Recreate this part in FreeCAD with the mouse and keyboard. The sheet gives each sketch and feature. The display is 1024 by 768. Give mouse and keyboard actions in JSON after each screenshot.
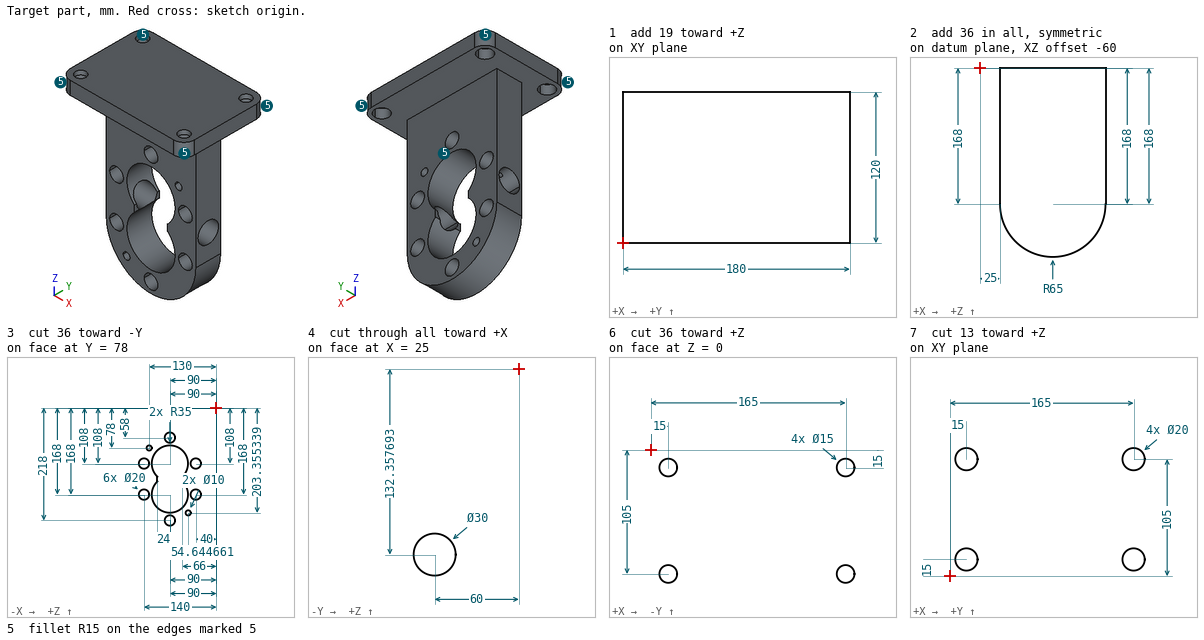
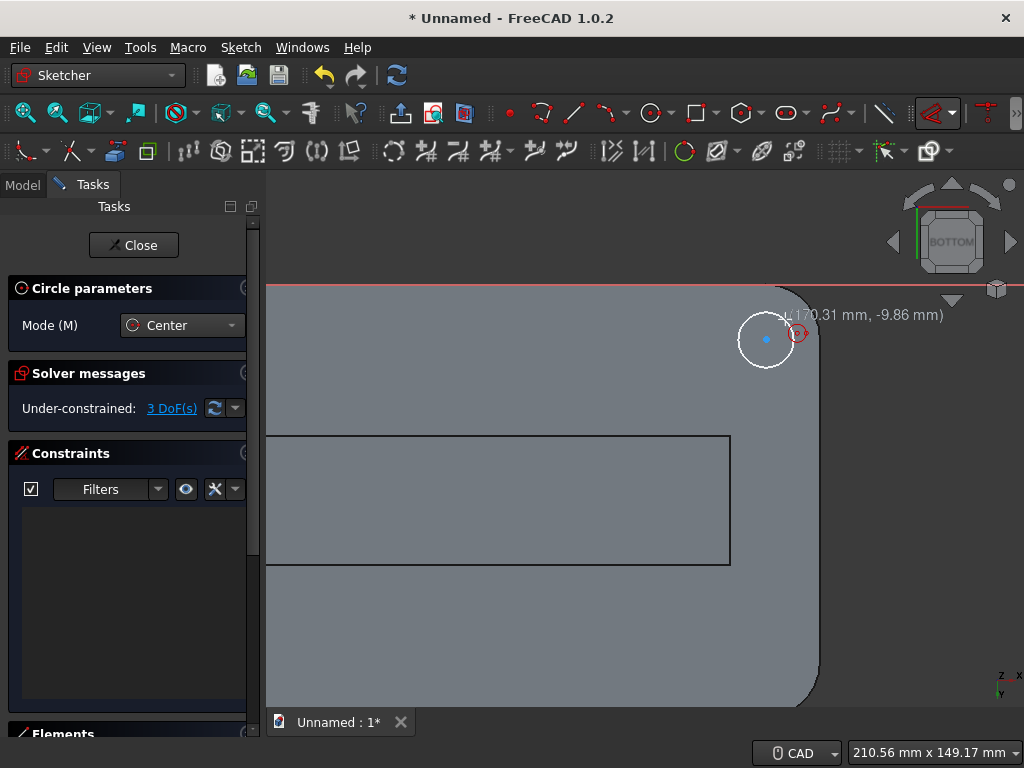
{"action": "scroll", "coordinate": [768, 340], "scroll_direction": "down", "scroll_amount": 2}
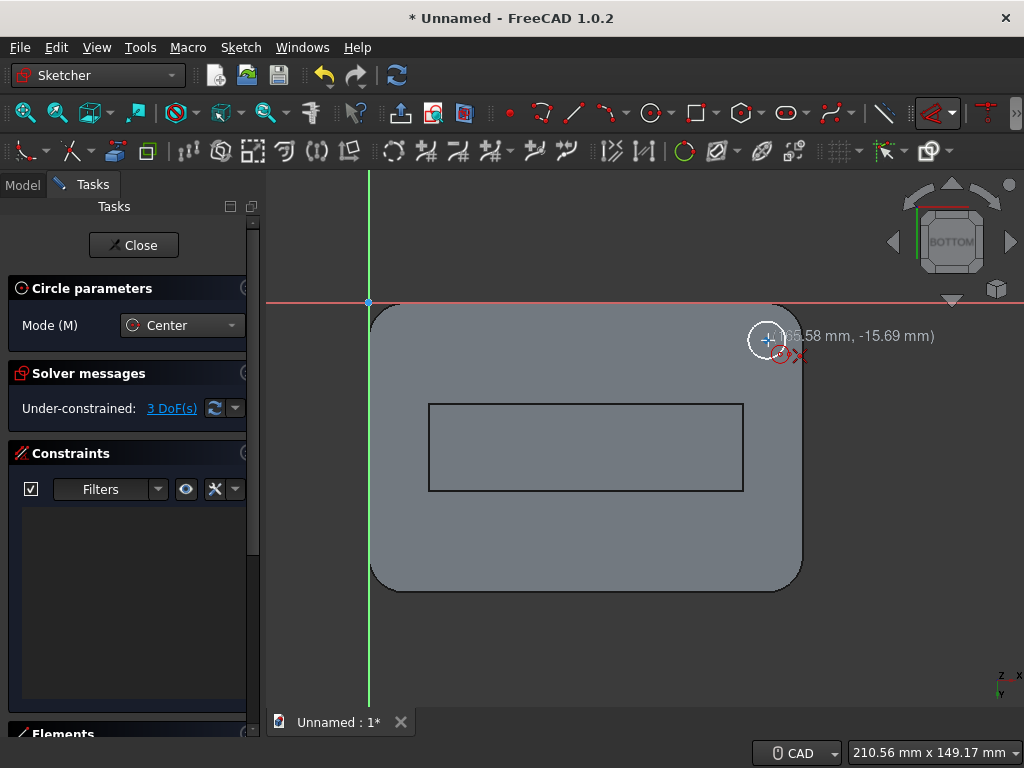
{"action": "scroll", "coordinate": [405, 339], "scroll_direction": "up", "scroll_amount": 2}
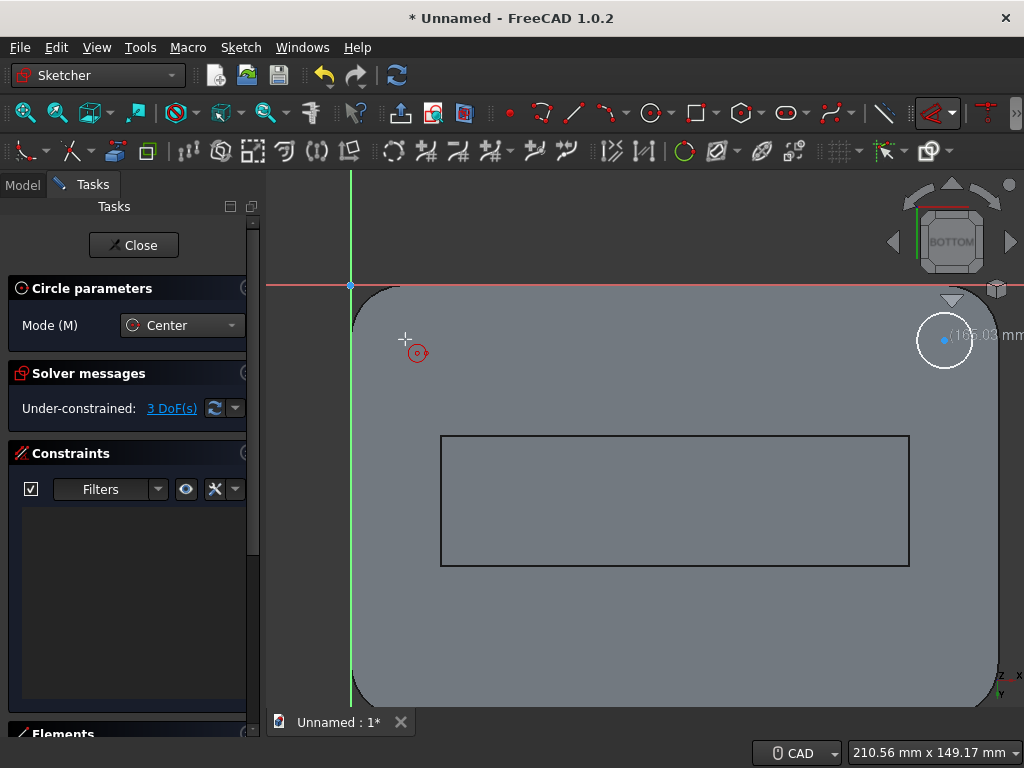
{"action": "left_click", "coordinate": [405, 339]}
{"action": "left_click", "coordinate": [424, 320]}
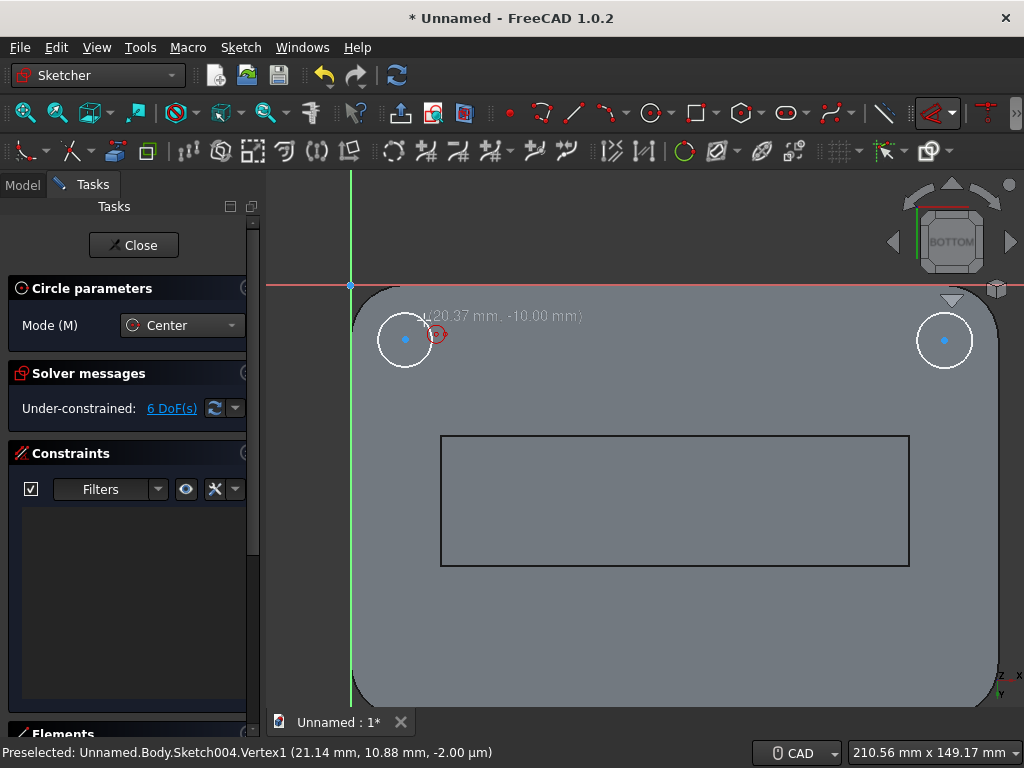
{"action": "left_click", "coordinate": [405, 663]}
{"action": "left_click", "coordinate": [424, 644]}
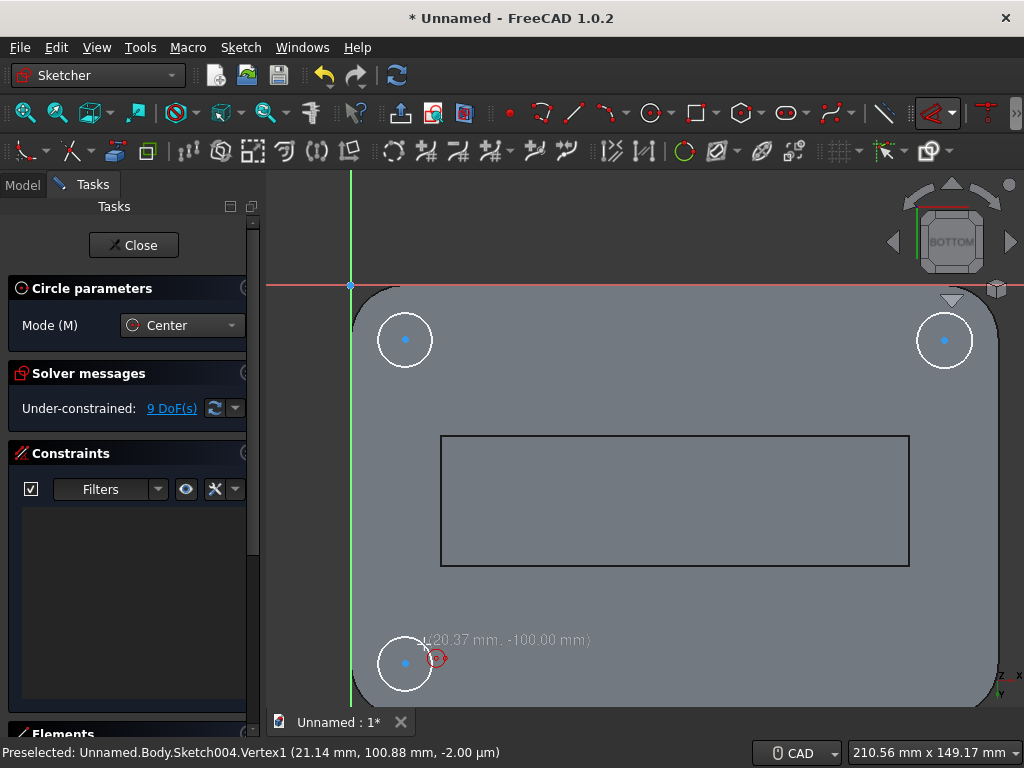
{"action": "scroll", "coordinate": [404, 339], "scroll_direction": "down", "scroll_amount": 2}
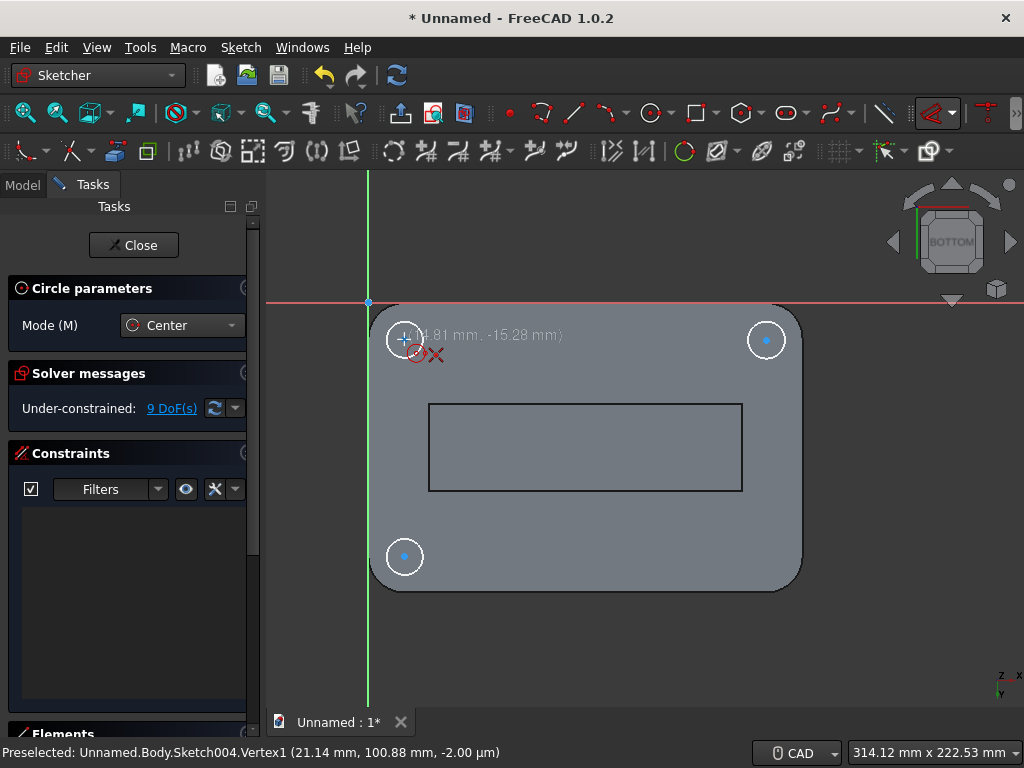
{"action": "scroll", "coordinate": [766, 556], "scroll_direction": "up", "scroll_amount": 2}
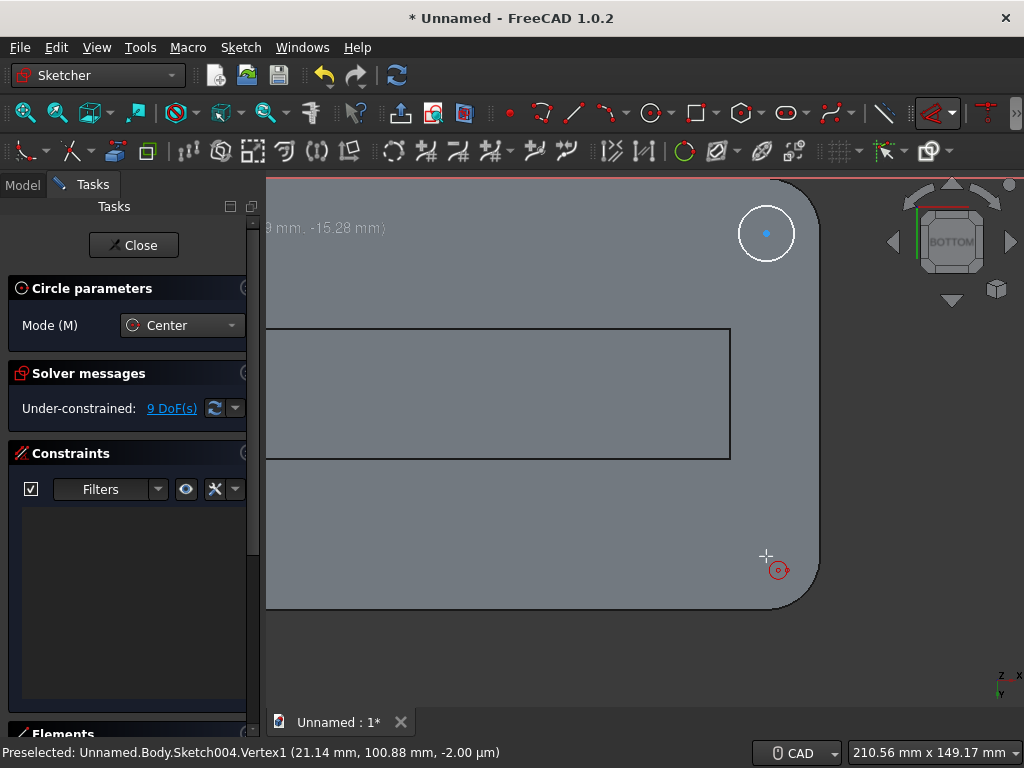
{"action": "left_click", "coordinate": [766, 556]}
{"action": "left_click", "coordinate": [785, 537]}
{"action": "key", "text": "Escape"}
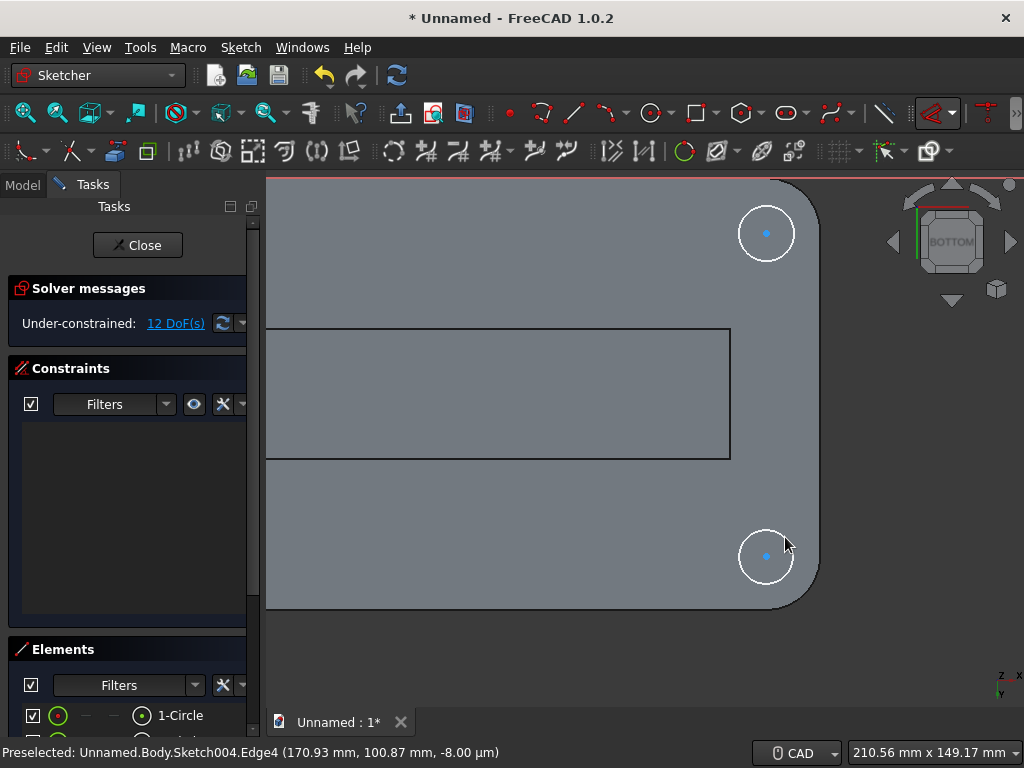
{"action": "left_click", "coordinate": [786, 214]}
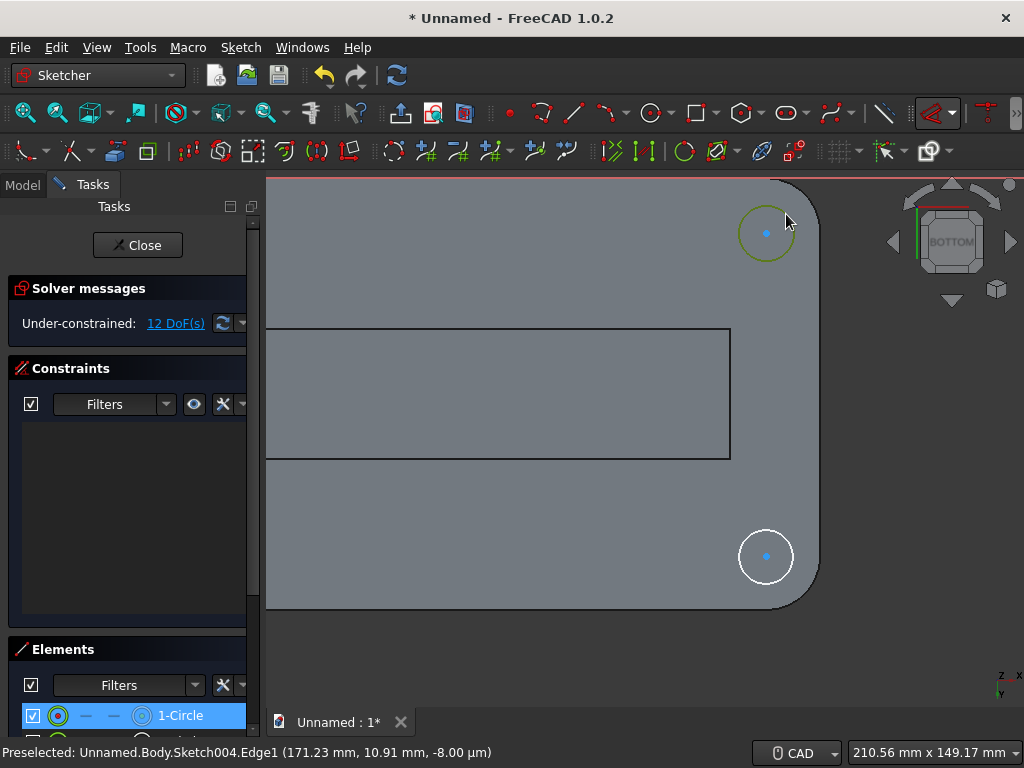
{"action": "scroll", "coordinate": [767, 556], "scroll_direction": "down", "scroll_amount": 2}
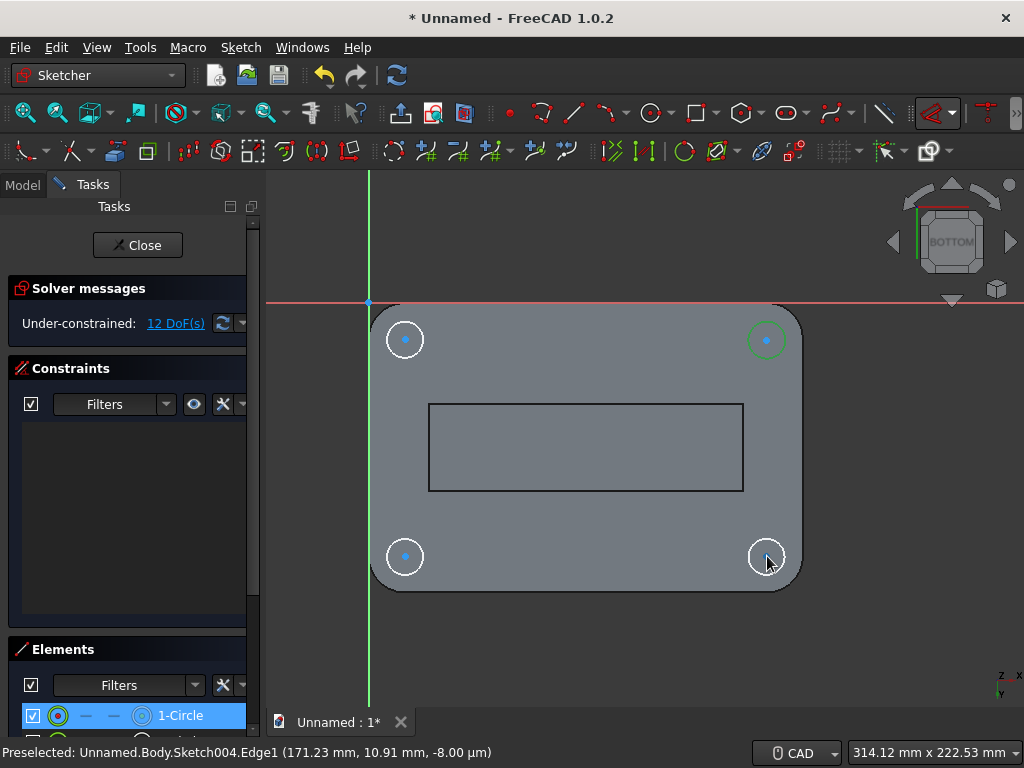
{"action": "left_click", "coordinate": [418, 327]}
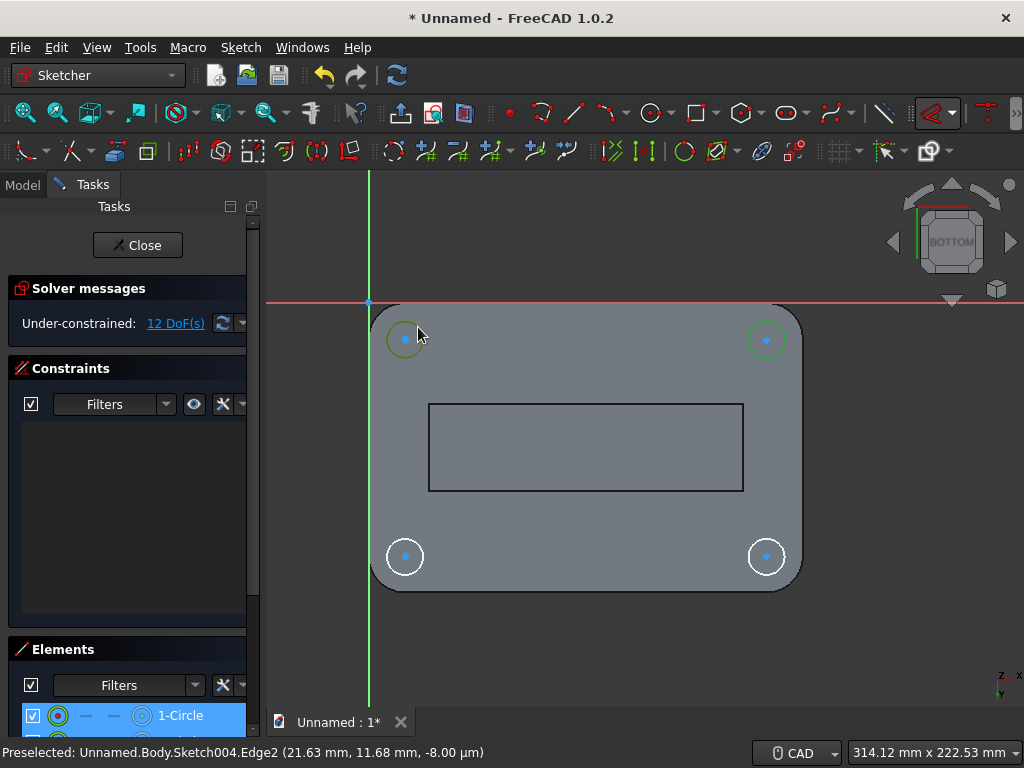
{"action": "left_click", "coordinate": [418, 544]}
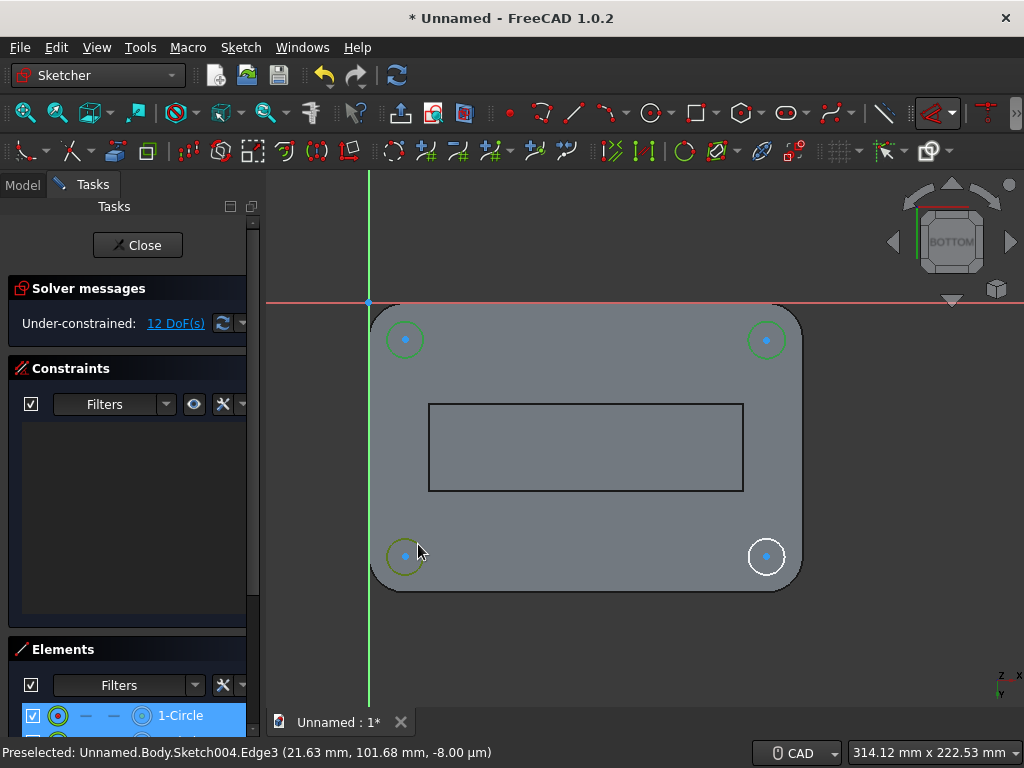
{"action": "left_click", "coordinate": [779, 544]}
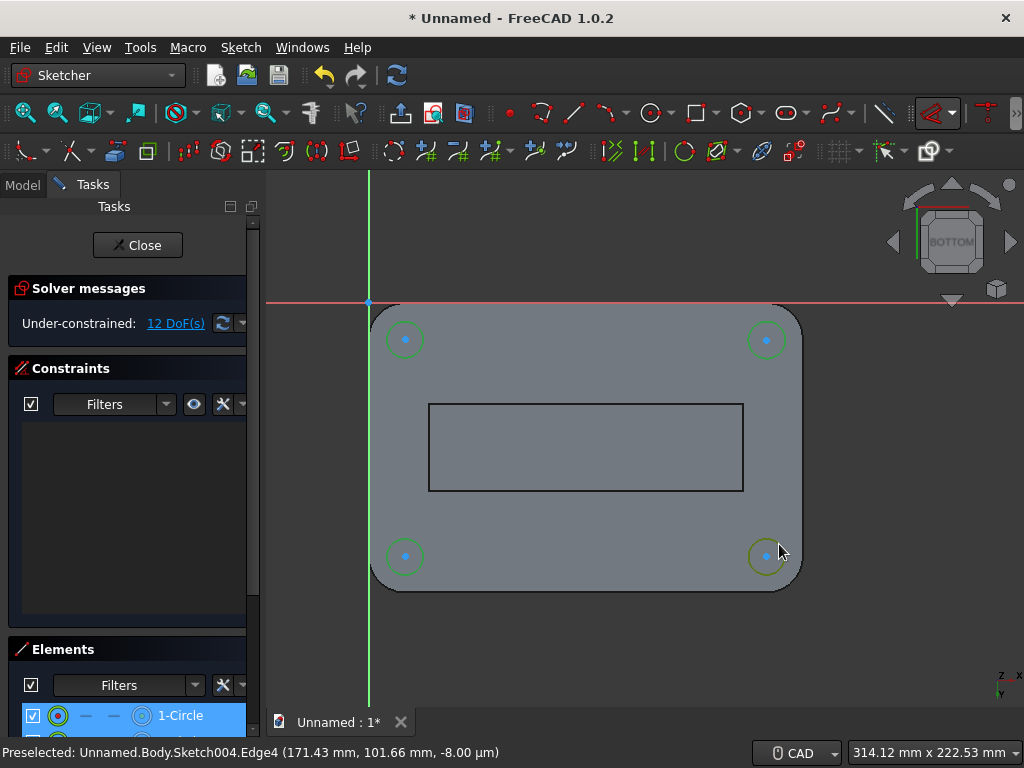
{"action": "key", "text": "e"}